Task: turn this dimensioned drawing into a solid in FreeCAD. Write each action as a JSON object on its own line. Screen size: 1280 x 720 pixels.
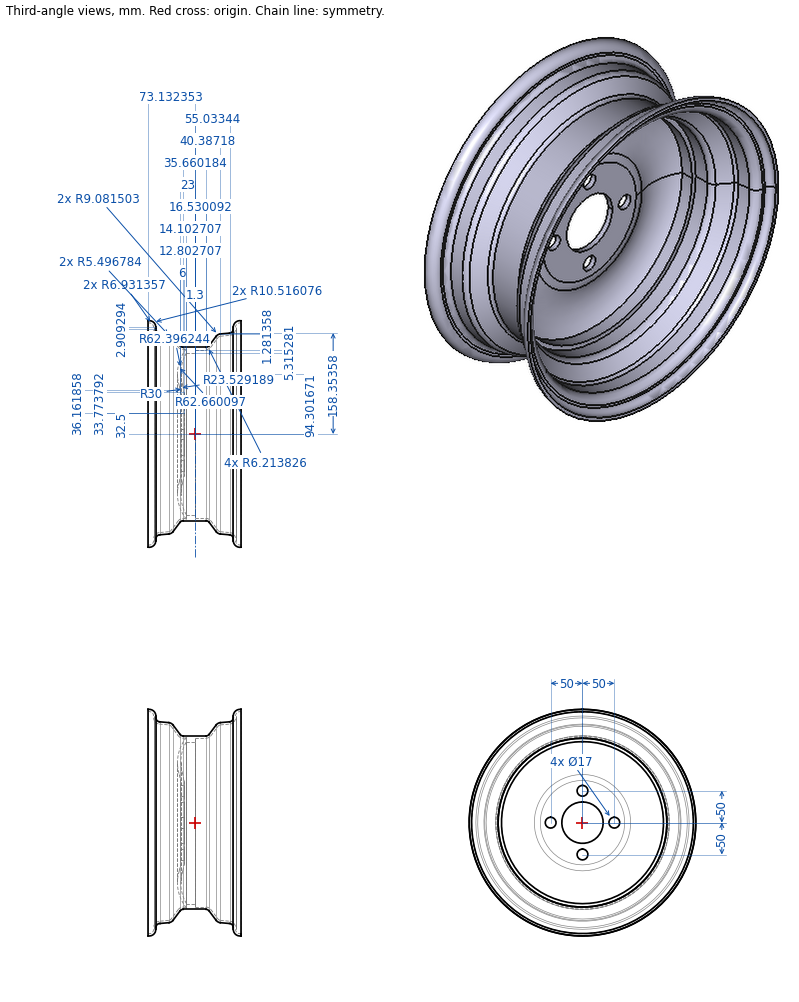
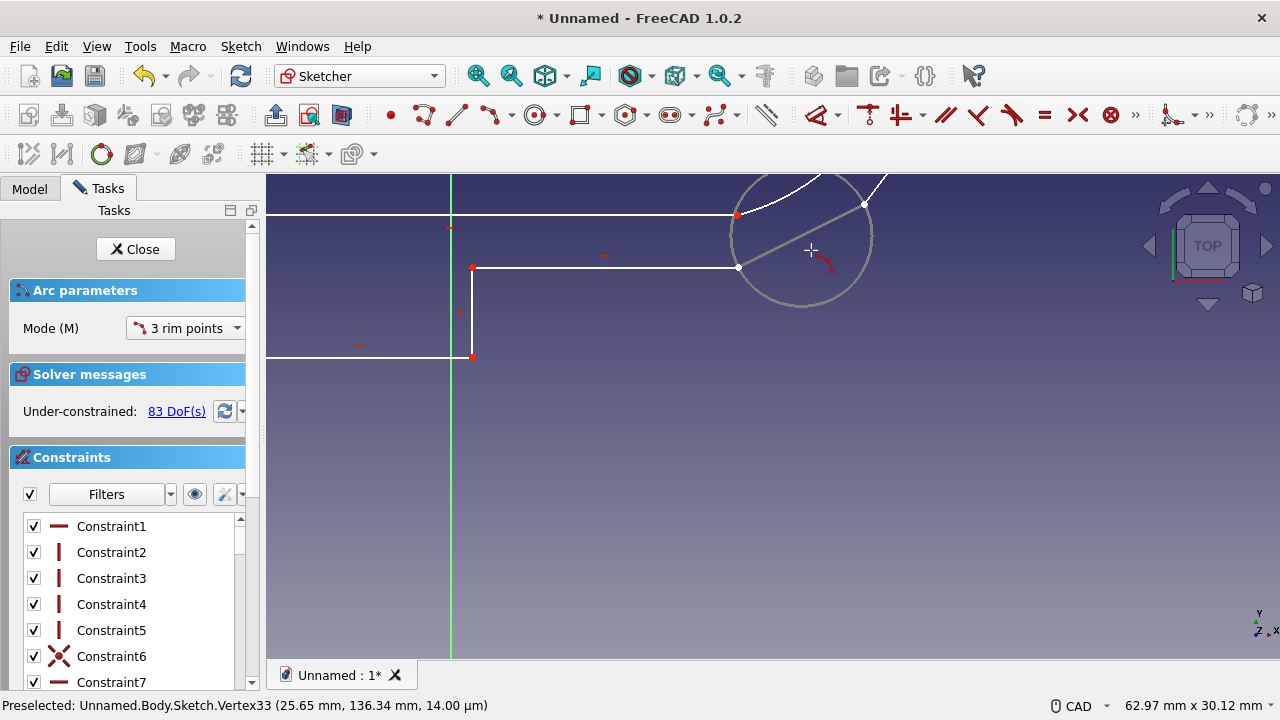
{"action": "left_click", "coordinate": [809, 249]}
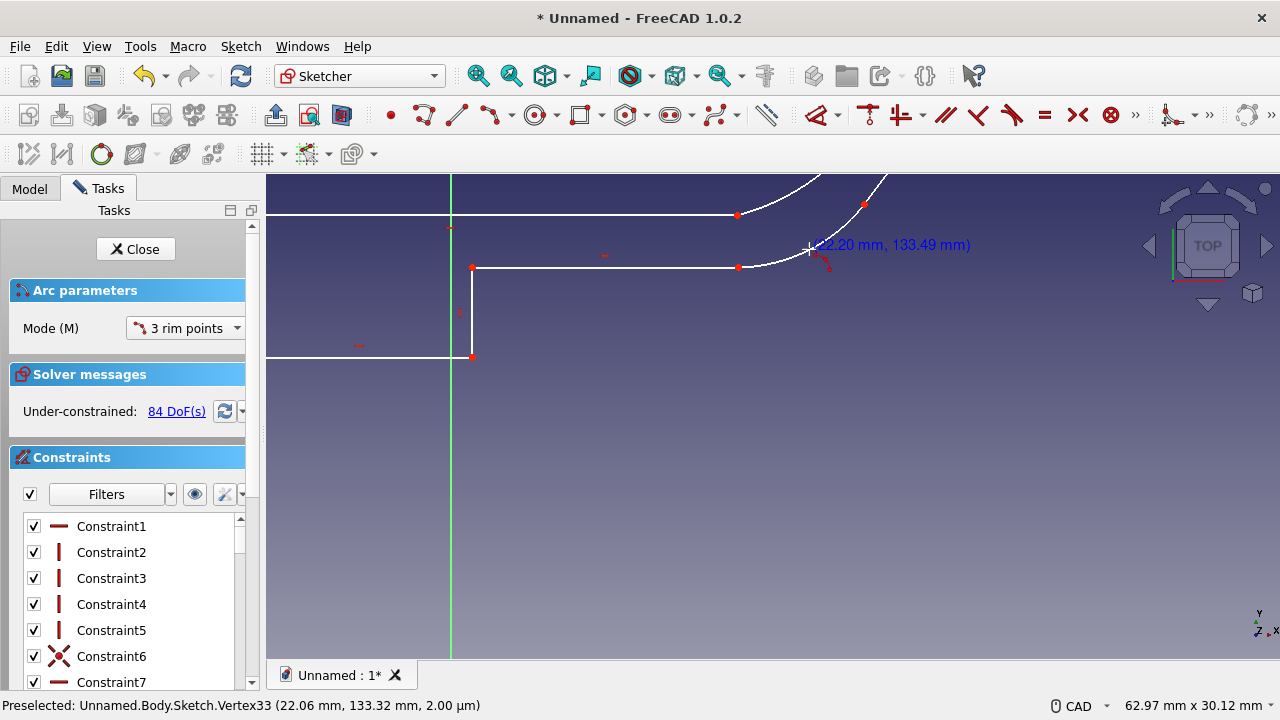
{"action": "scroll", "coordinate": [736, 348], "scroll_direction": "down", "scroll_amount": 11}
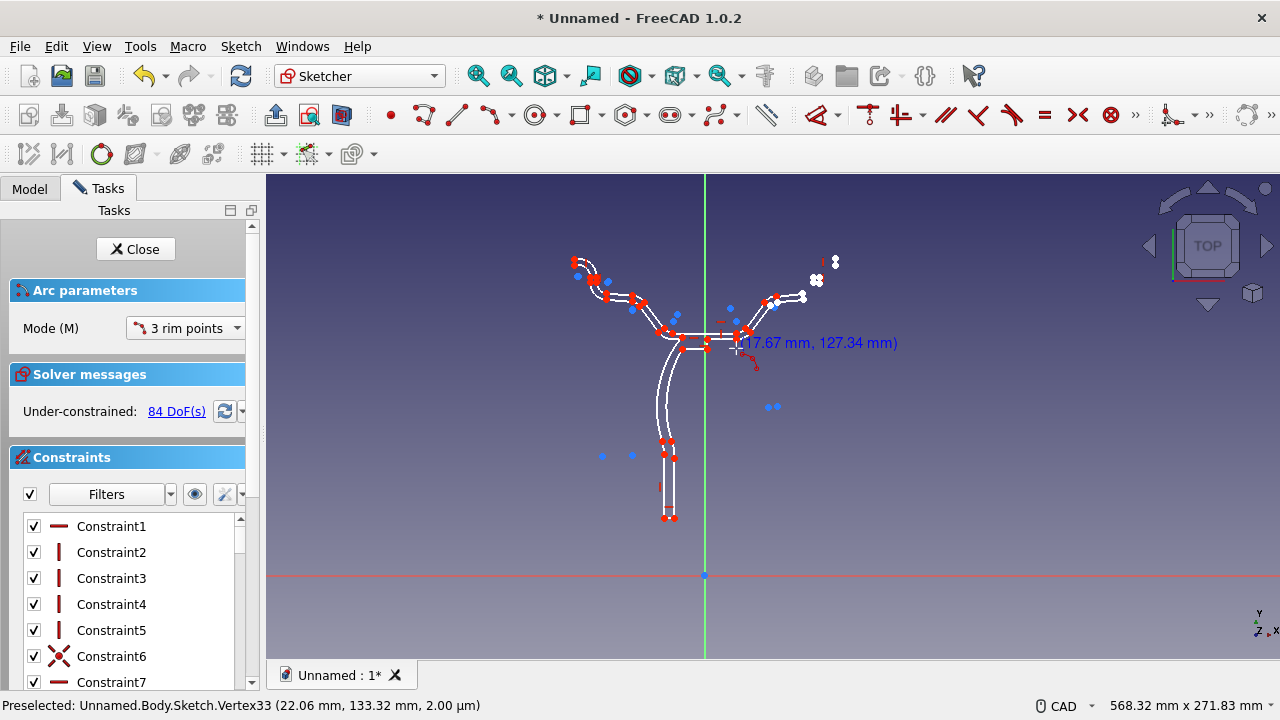
{"action": "scroll", "coordinate": [770, 306], "scroll_direction": "up", "scroll_amount": 5}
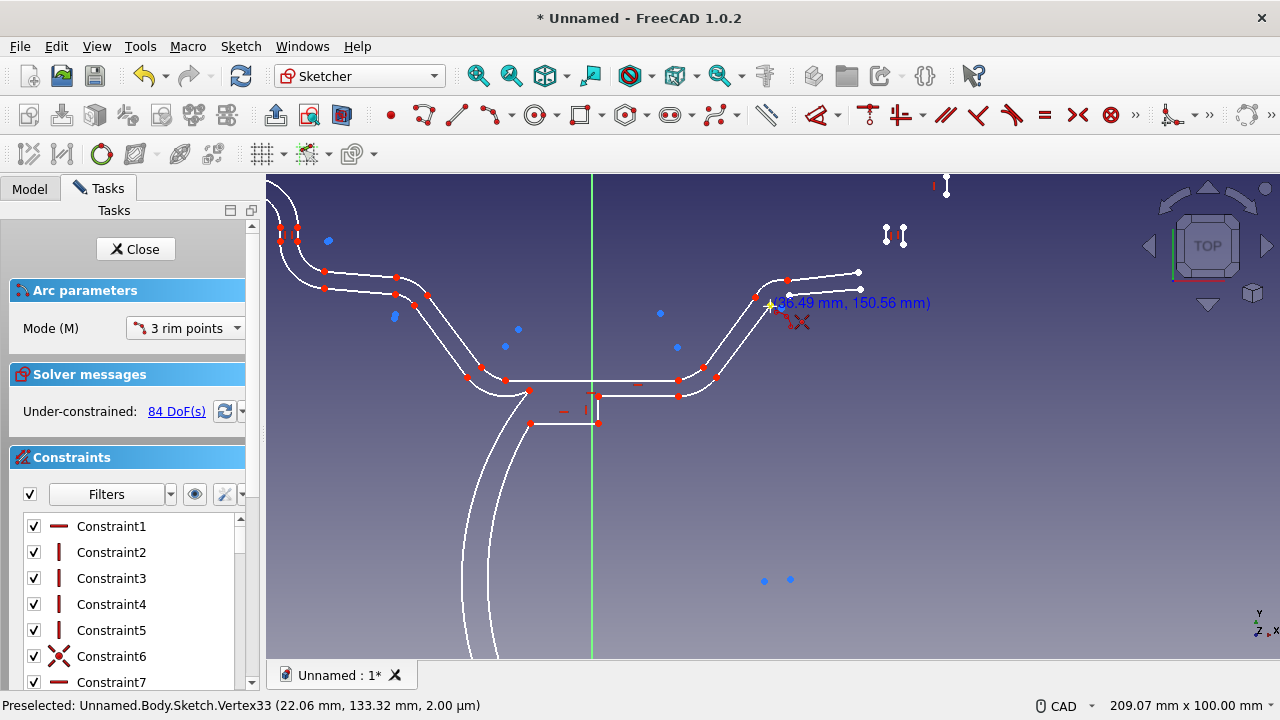
{"action": "left_click", "coordinate": [771, 305]}
{"action": "left_click", "coordinate": [790, 295]}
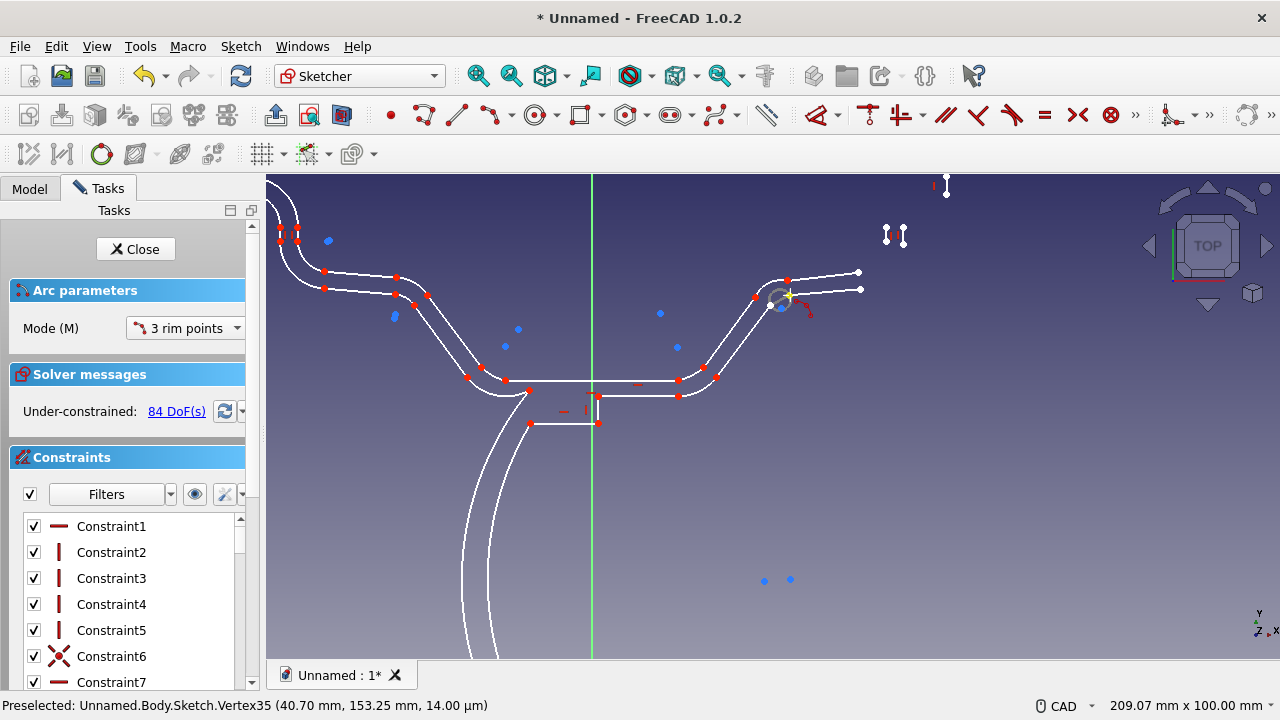
{"action": "scroll", "coordinate": [779, 297], "scroll_direction": "up", "scroll_amount": 10}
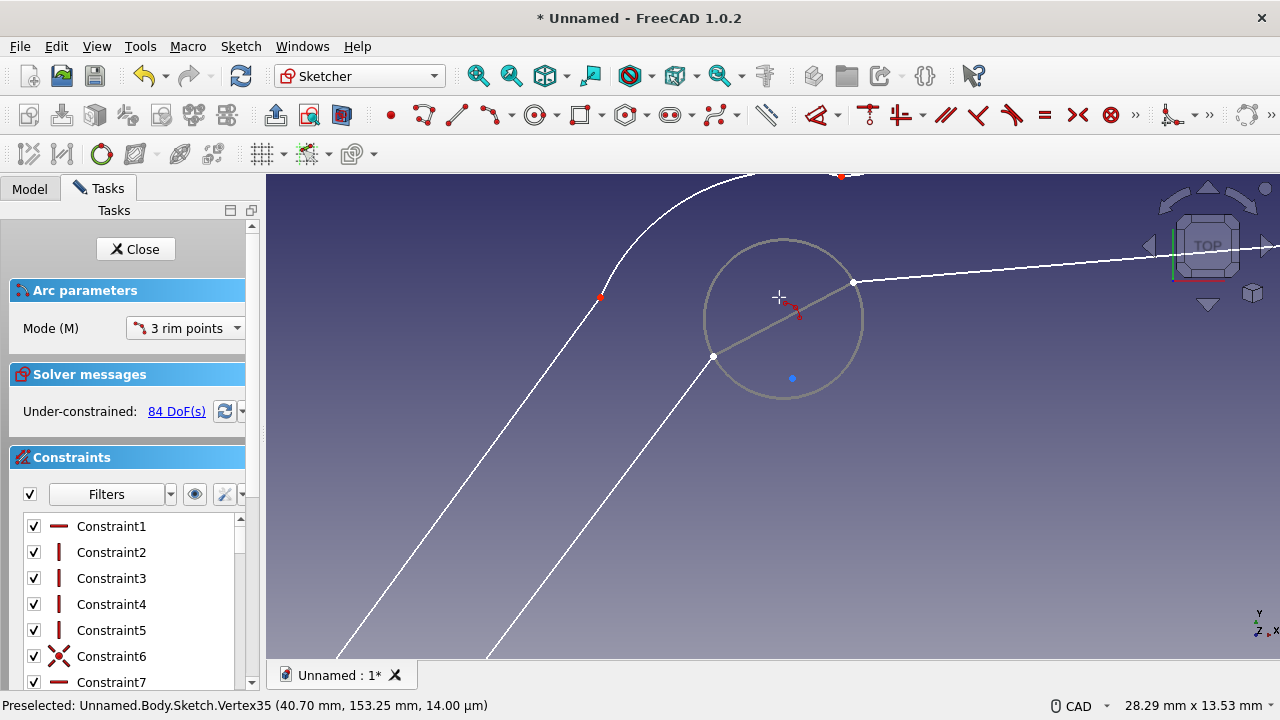
{"action": "left_click", "coordinate": [775, 297]}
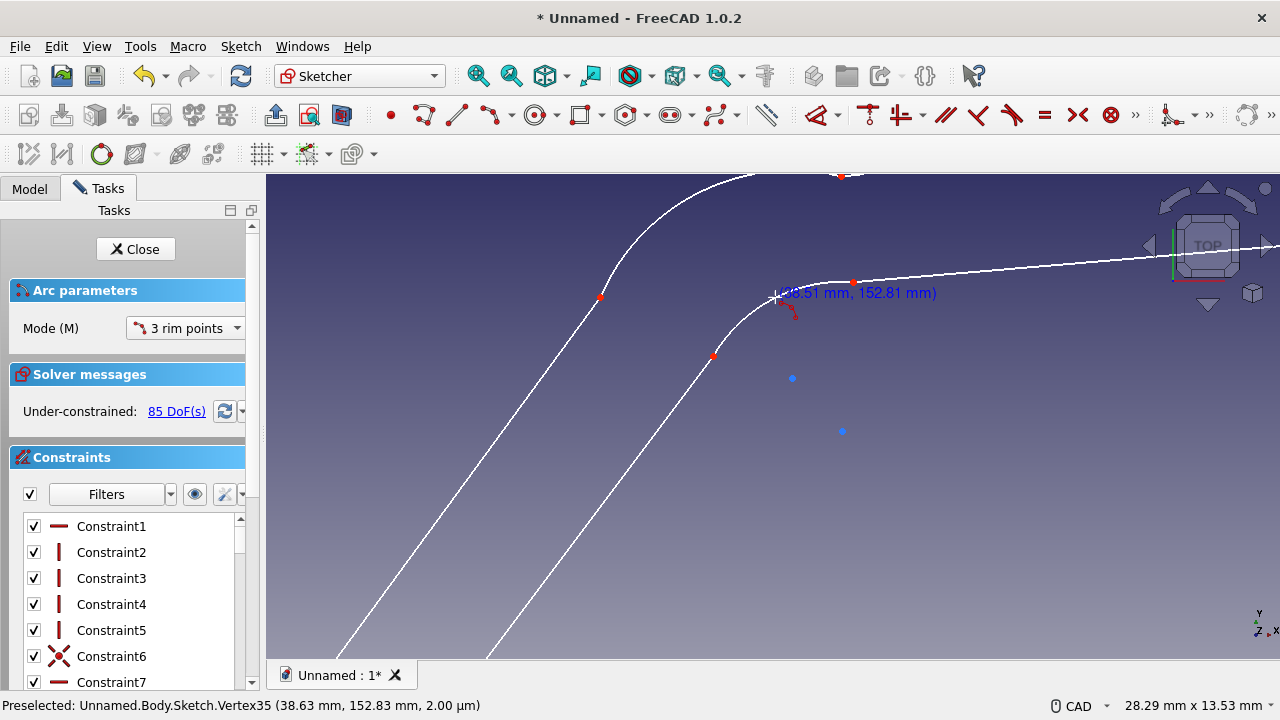
{"action": "scroll", "coordinate": [773, 303], "scroll_direction": "down", "scroll_amount": 15}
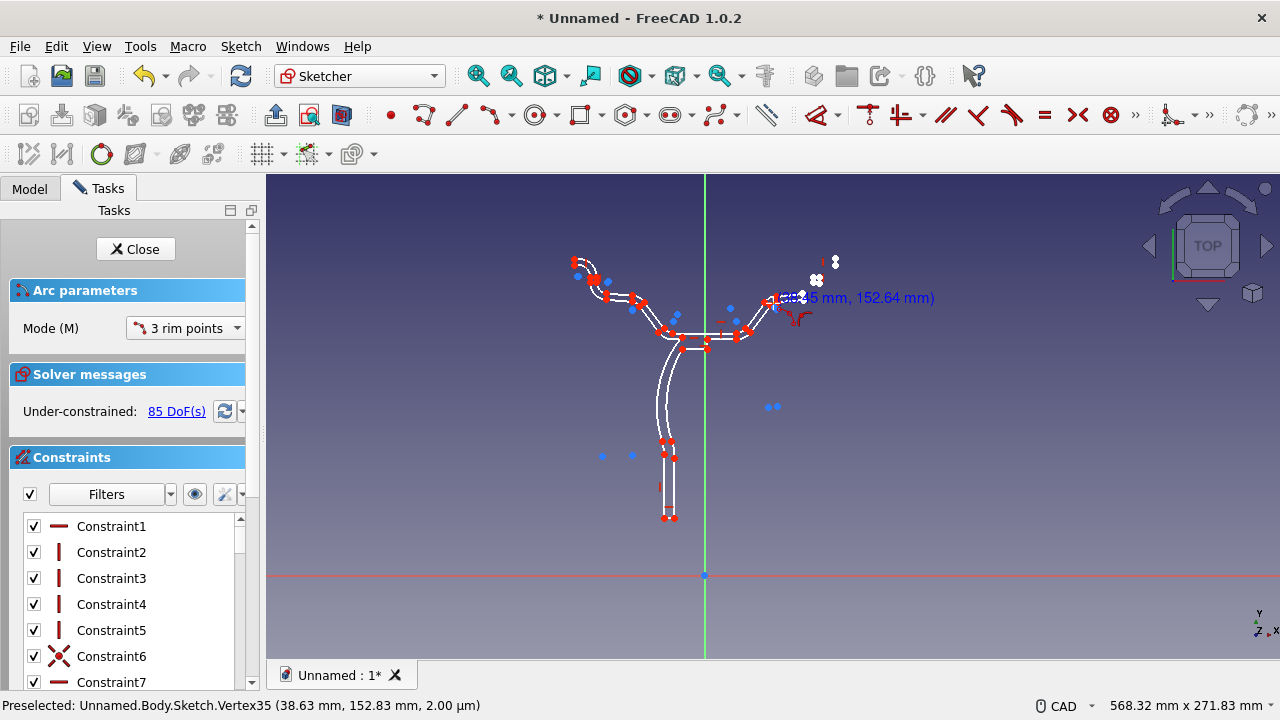
{"action": "scroll", "coordinate": [804, 299], "scroll_direction": "up", "scroll_amount": 5}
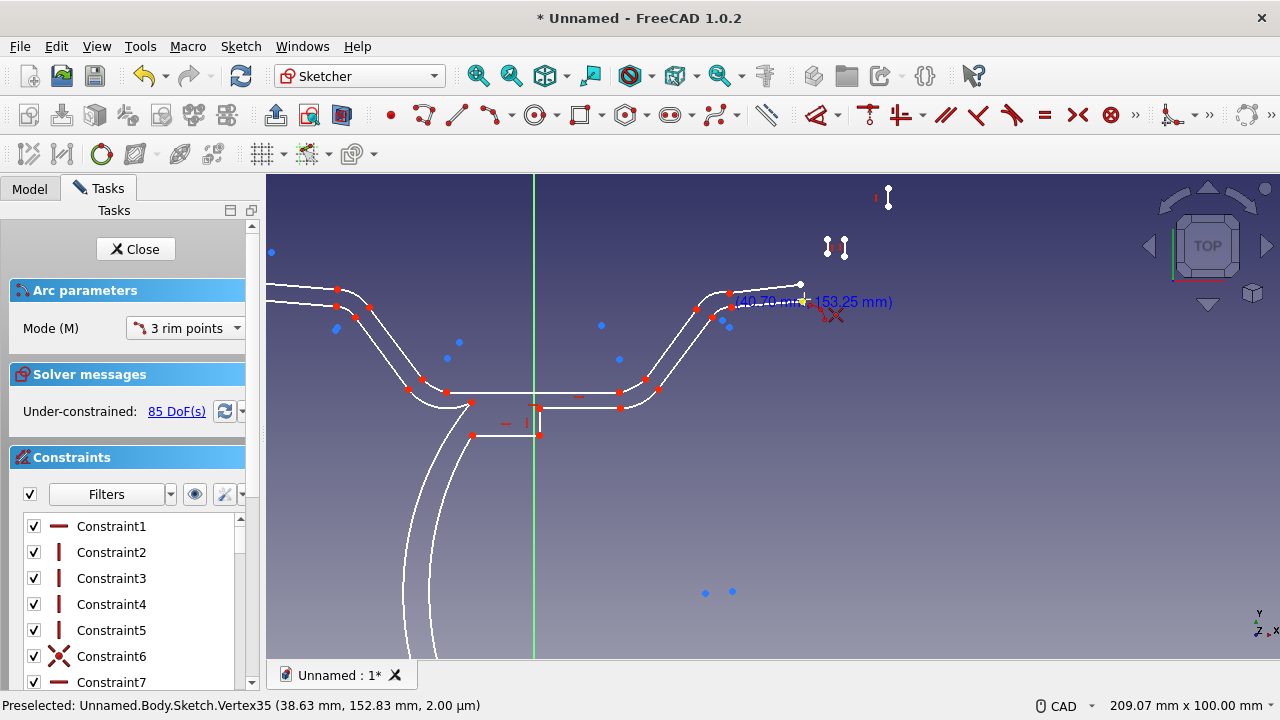
{"action": "left_click", "coordinate": [802, 301]}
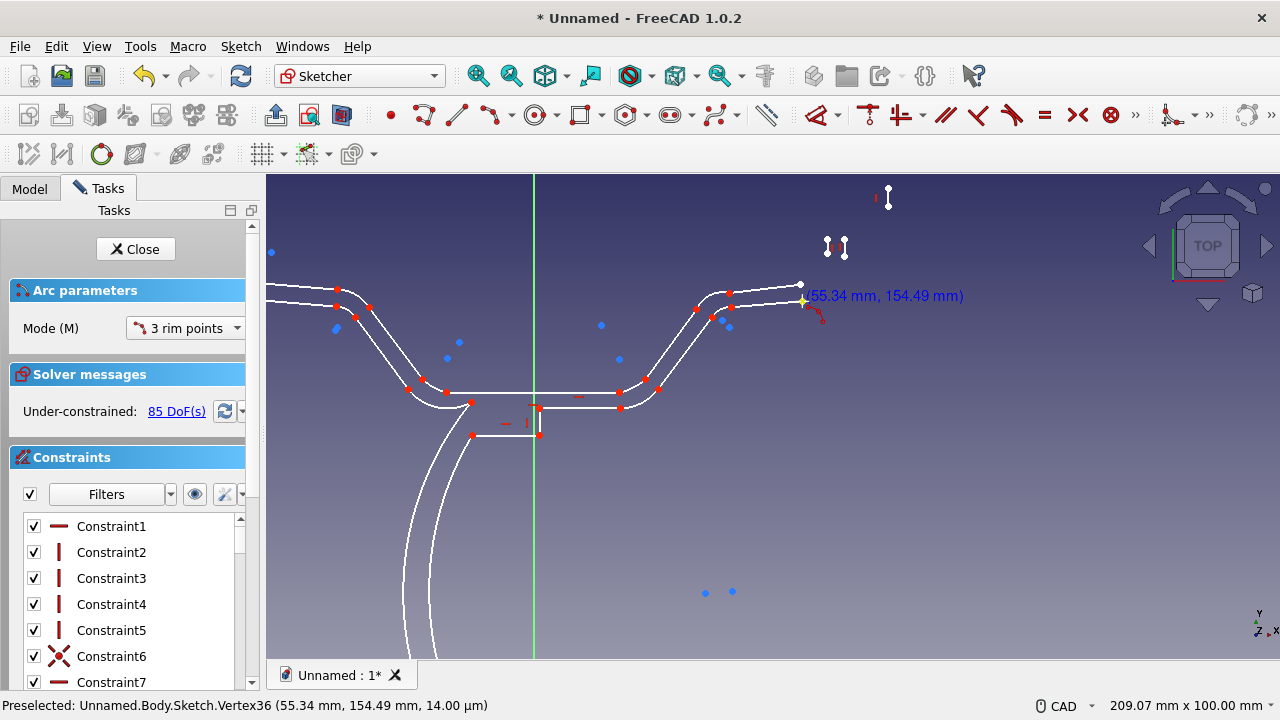
{"action": "scroll", "coordinate": [845, 253], "scroll_direction": "up", "scroll_amount": 5}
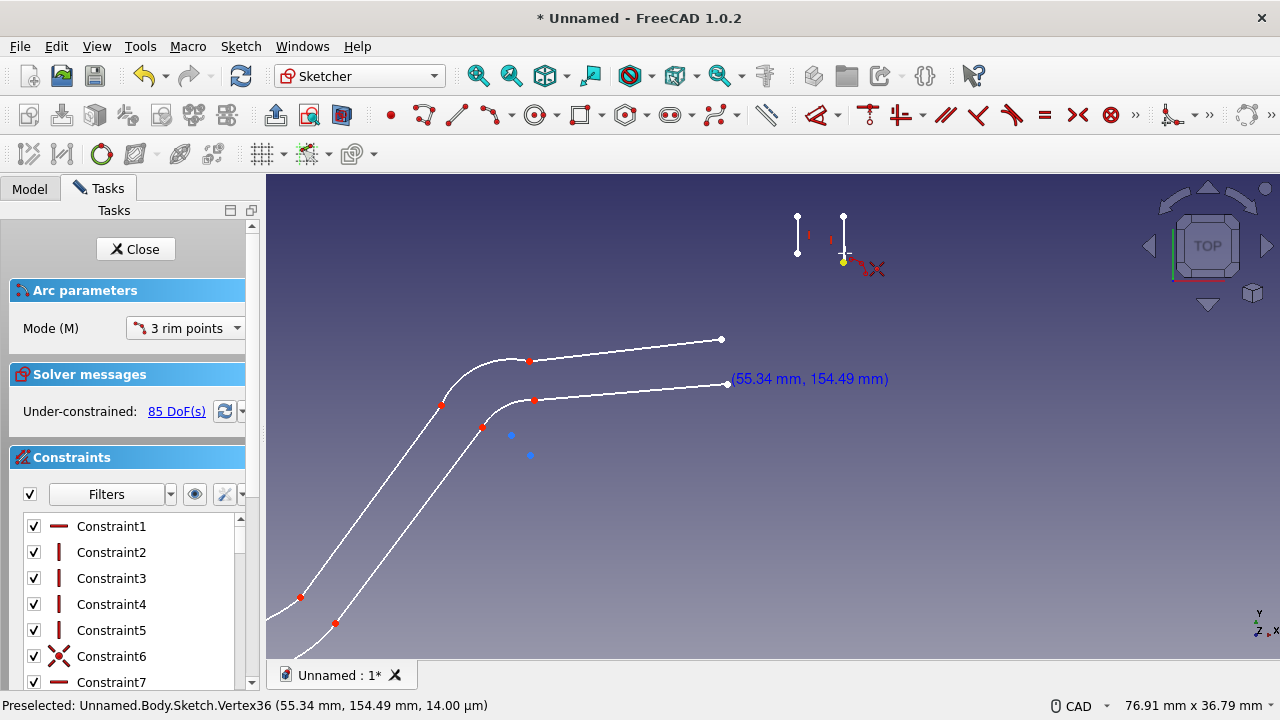
{"action": "left_click", "coordinate": [844, 262]}
{"action": "left_click", "coordinate": [811, 339]}